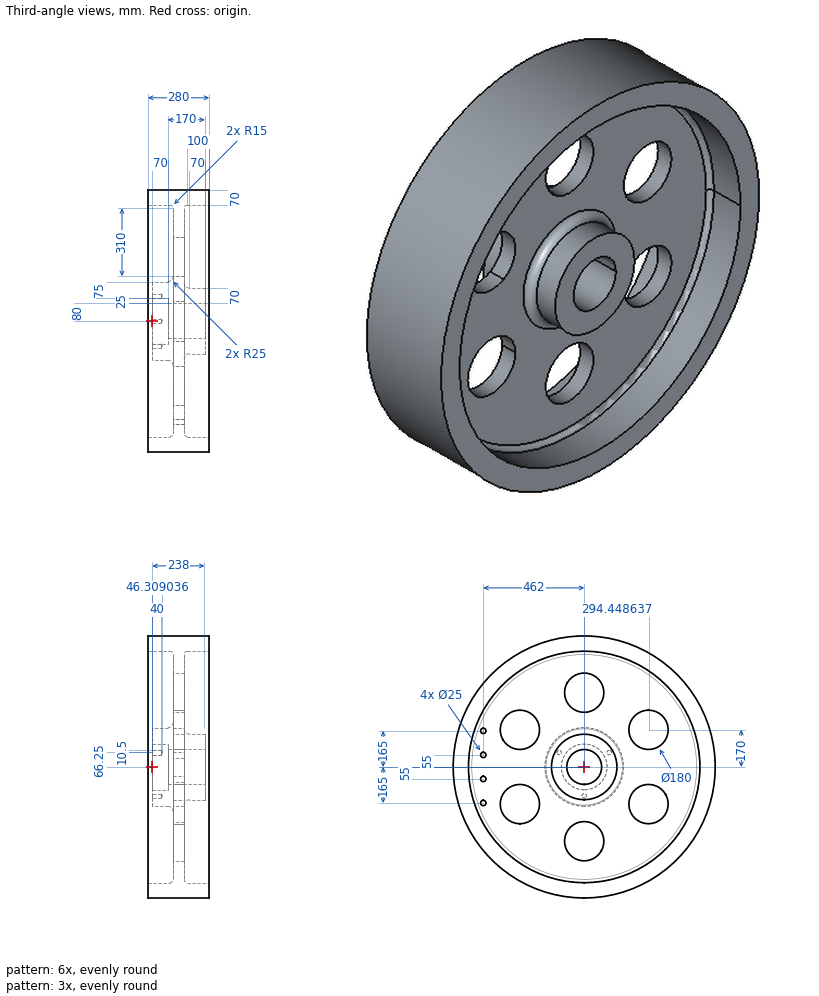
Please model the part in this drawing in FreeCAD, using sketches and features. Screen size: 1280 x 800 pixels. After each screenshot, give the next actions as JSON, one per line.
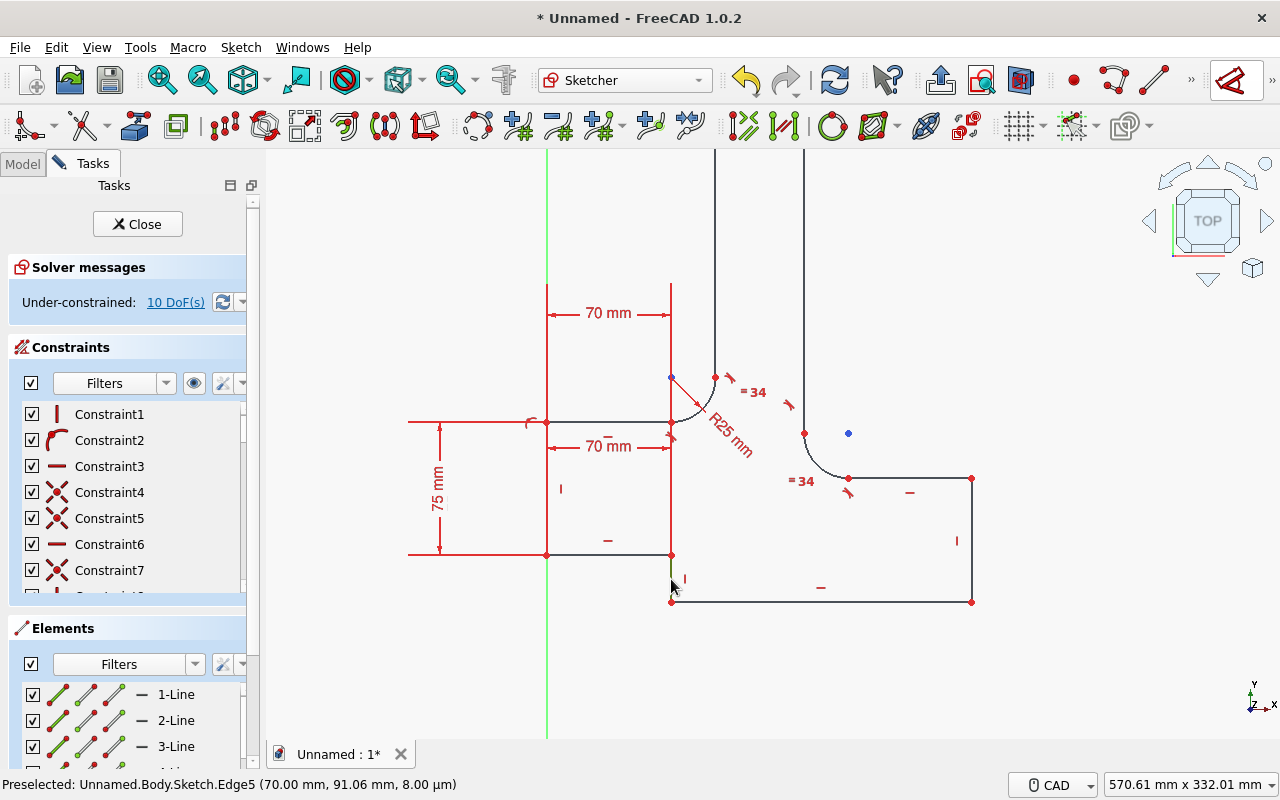
{"action": "key", "text": "i"}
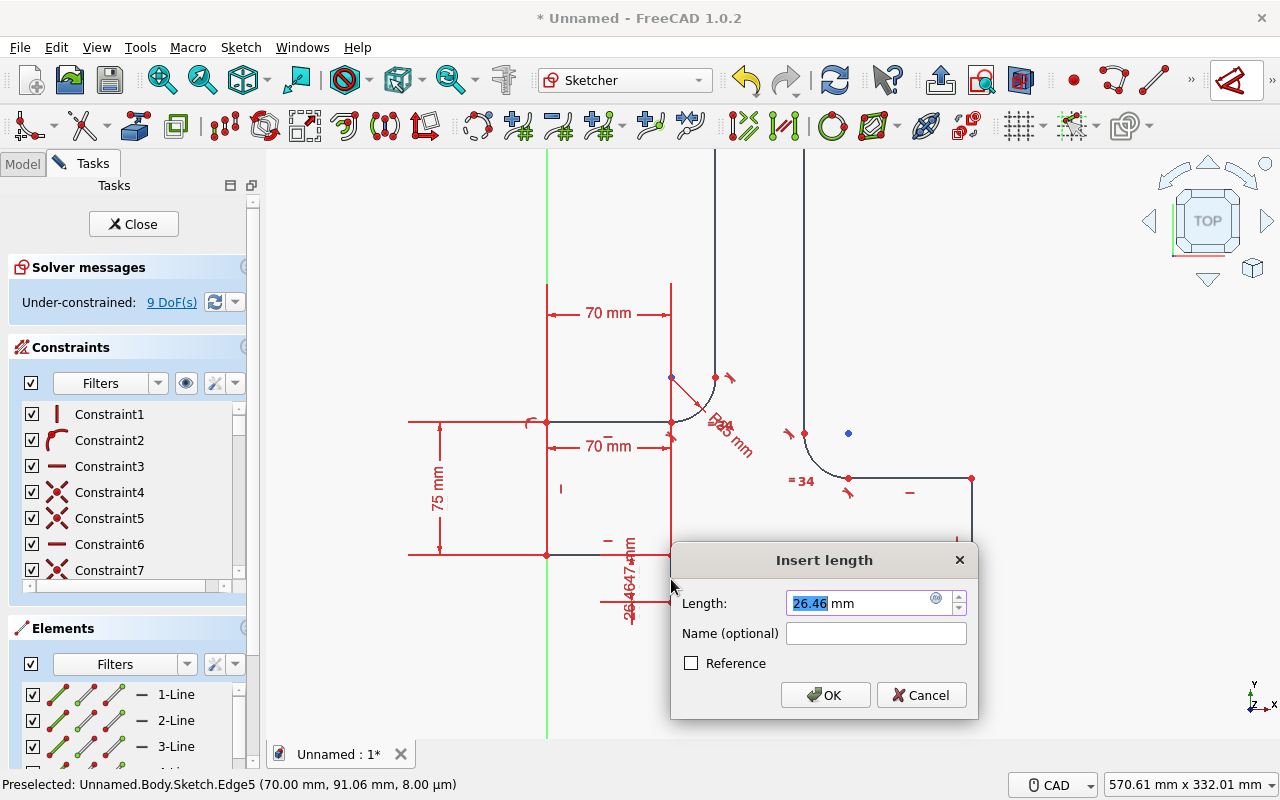
{"action": "type", "text": "25"}
{"action": "key", "text": "Return"}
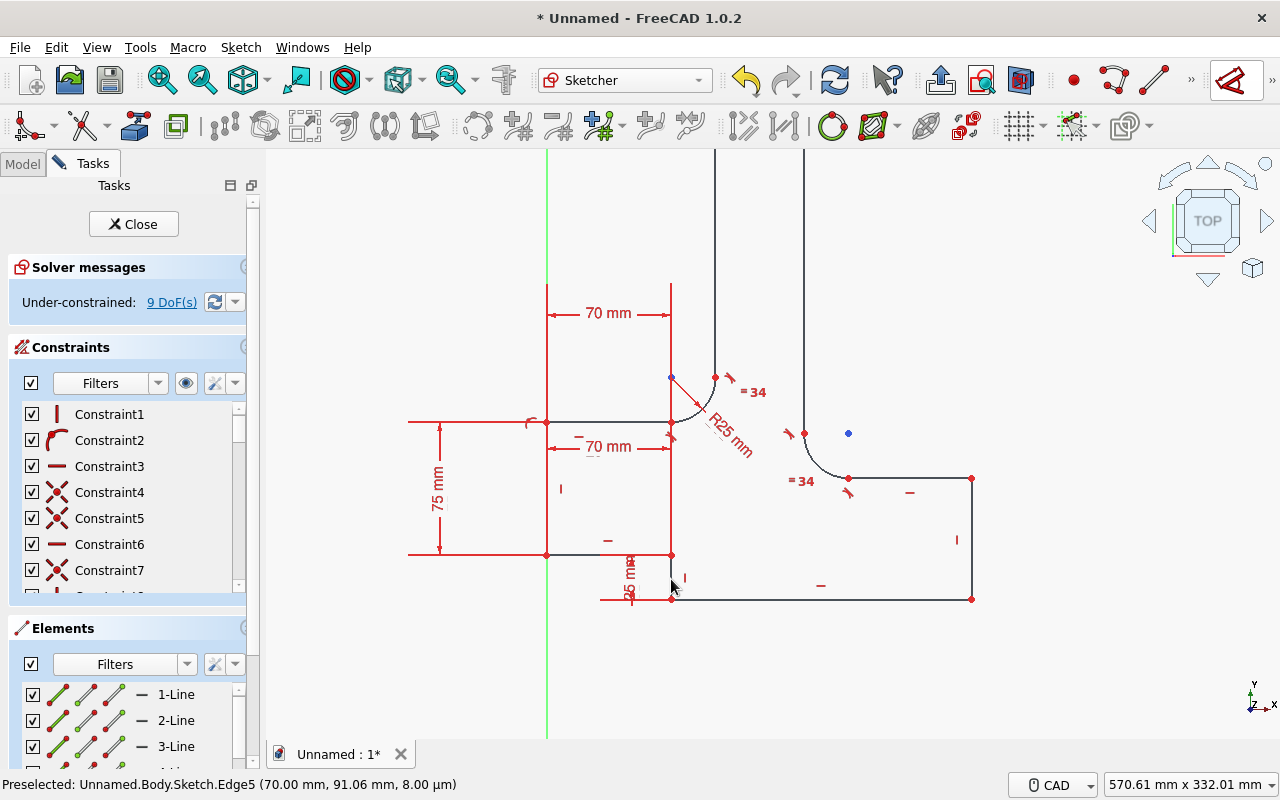
{"action": "left_click", "coordinate": [972, 563]}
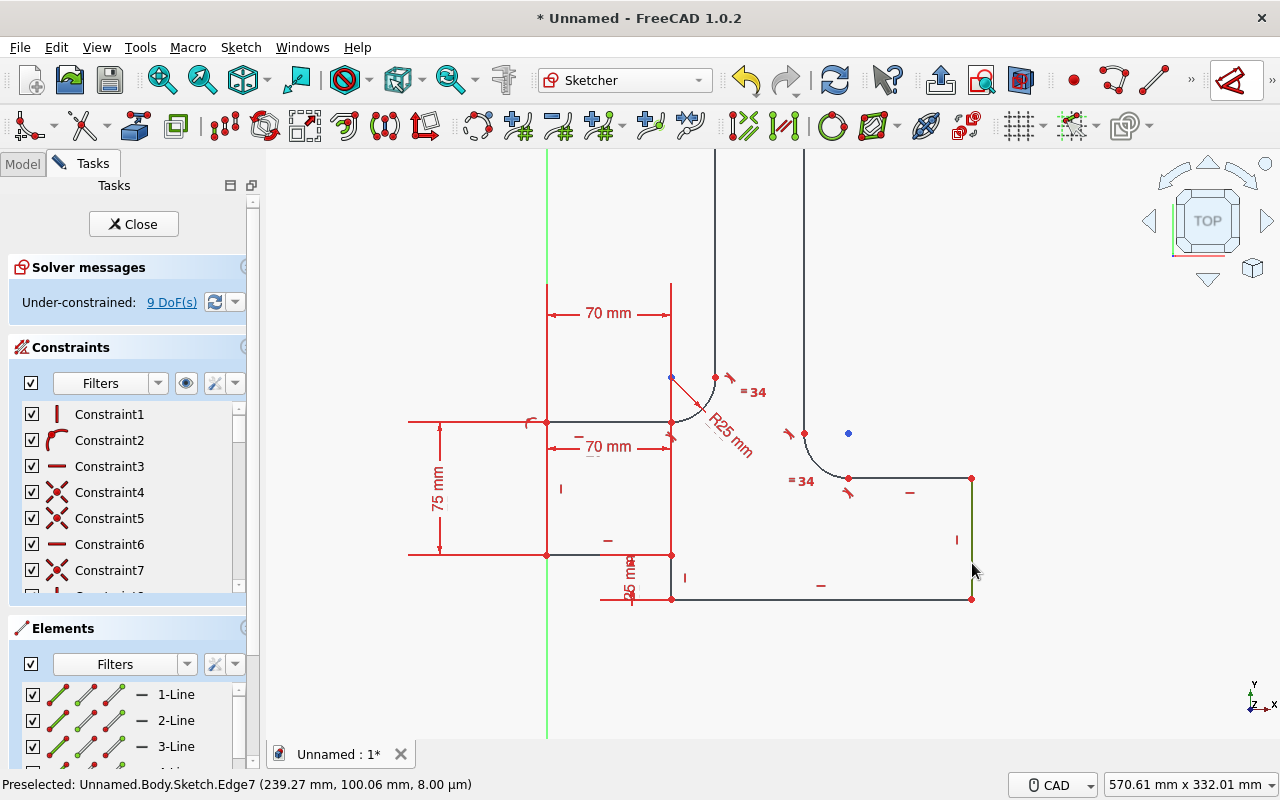
{"action": "left_click", "coordinate": [1258, 80]}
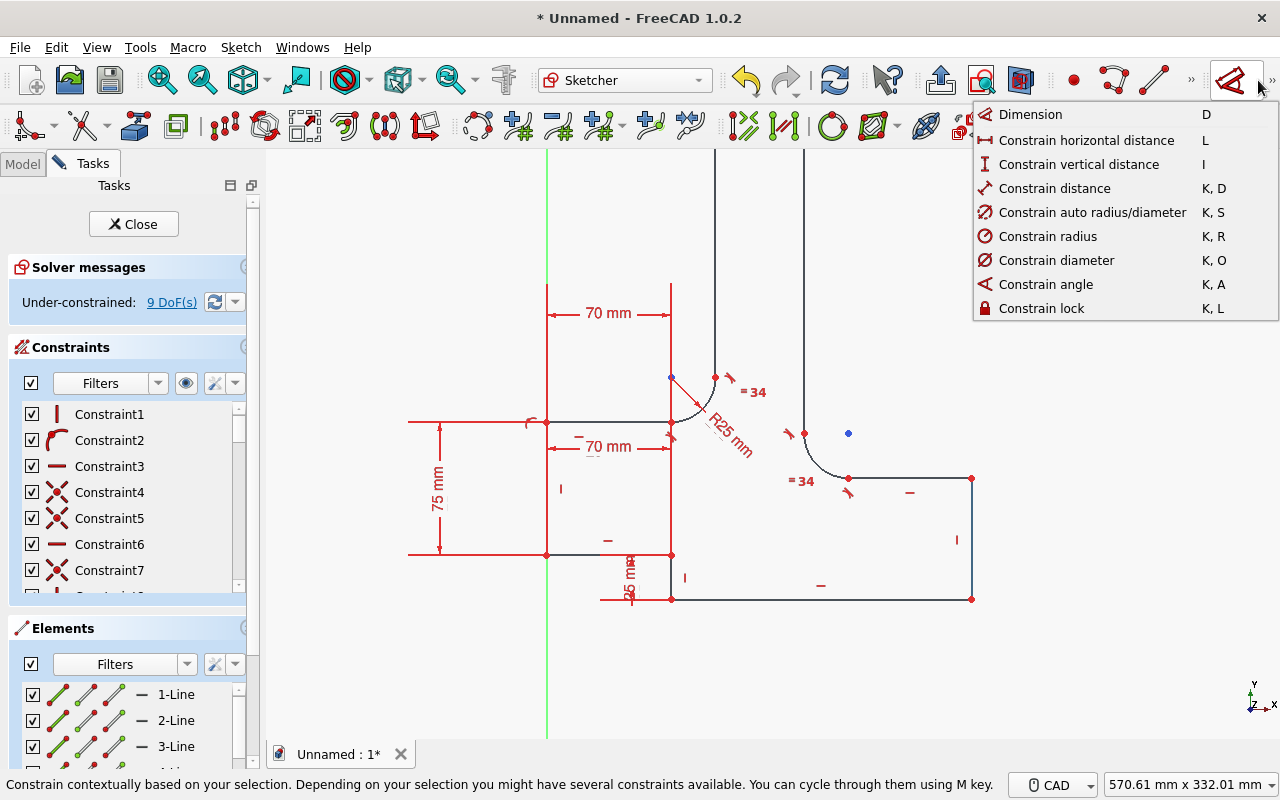
{"action": "left_click", "coordinate": [1126, 164]}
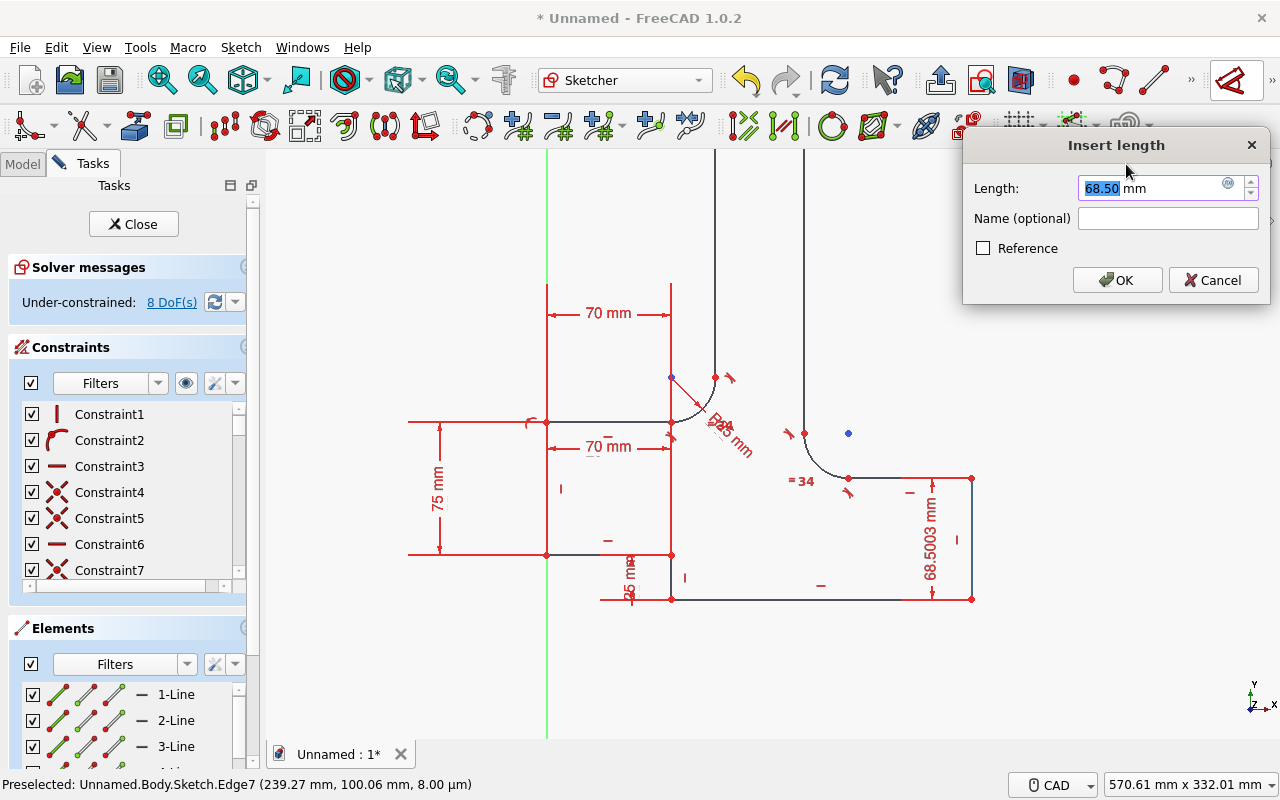
{"action": "type", "text": "70"}
{"action": "key", "text": "Return"}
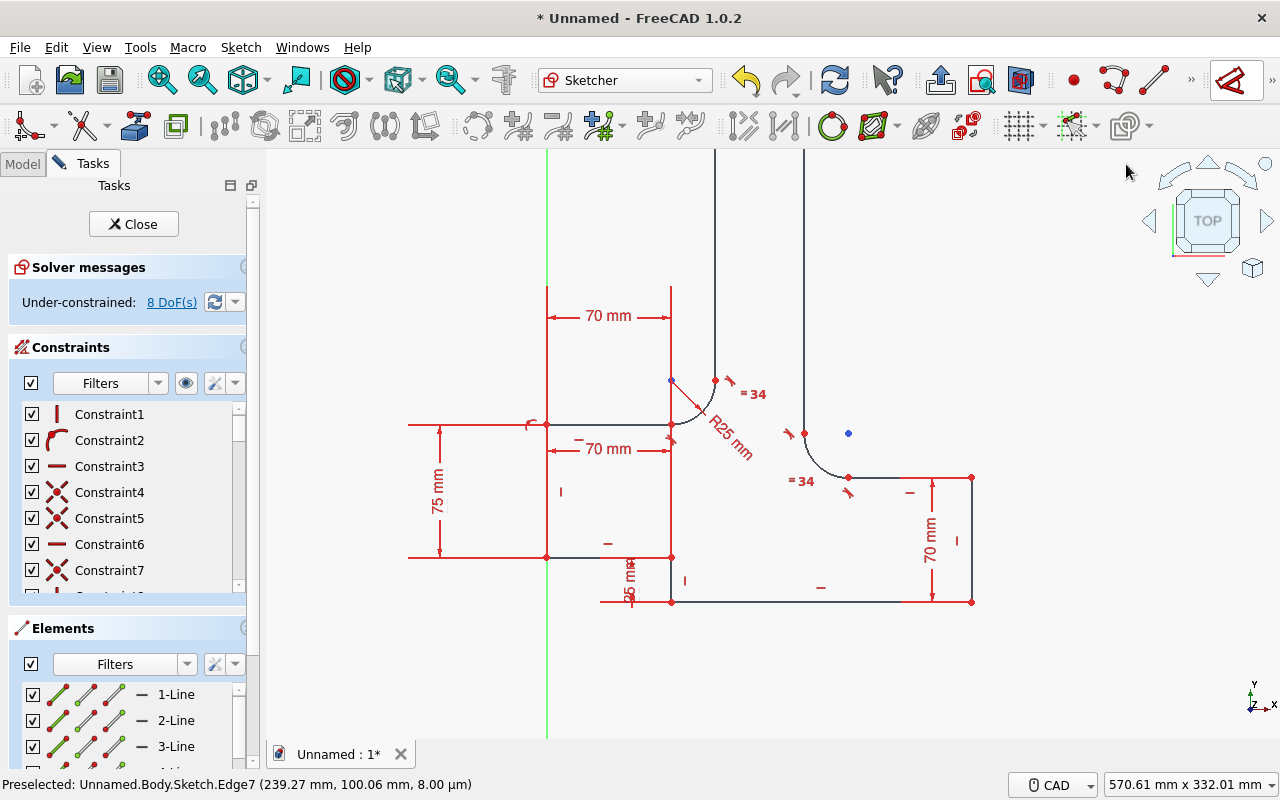
{"action": "left_click", "coordinate": [935, 478]}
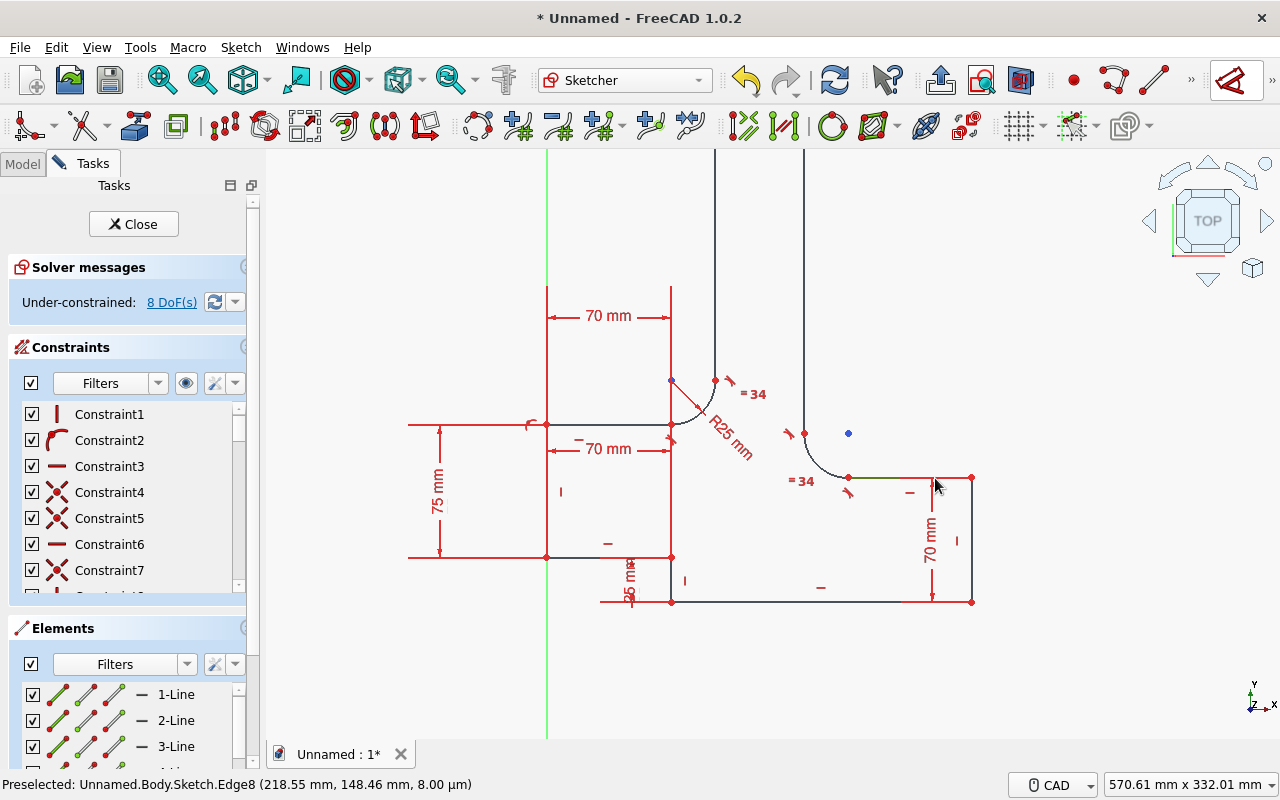
{"action": "key", "text": "l"}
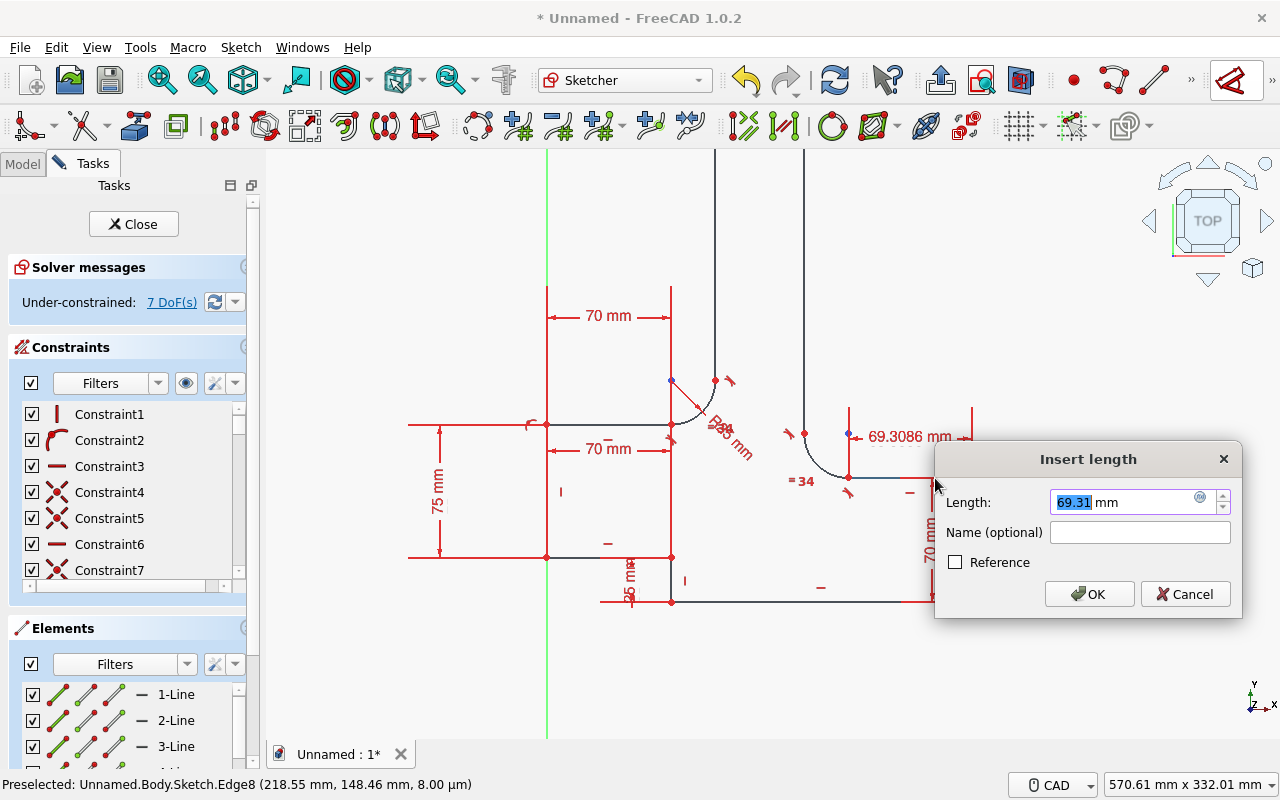
{"action": "type", "text": "70"}
{"action": "key", "text": "Return"}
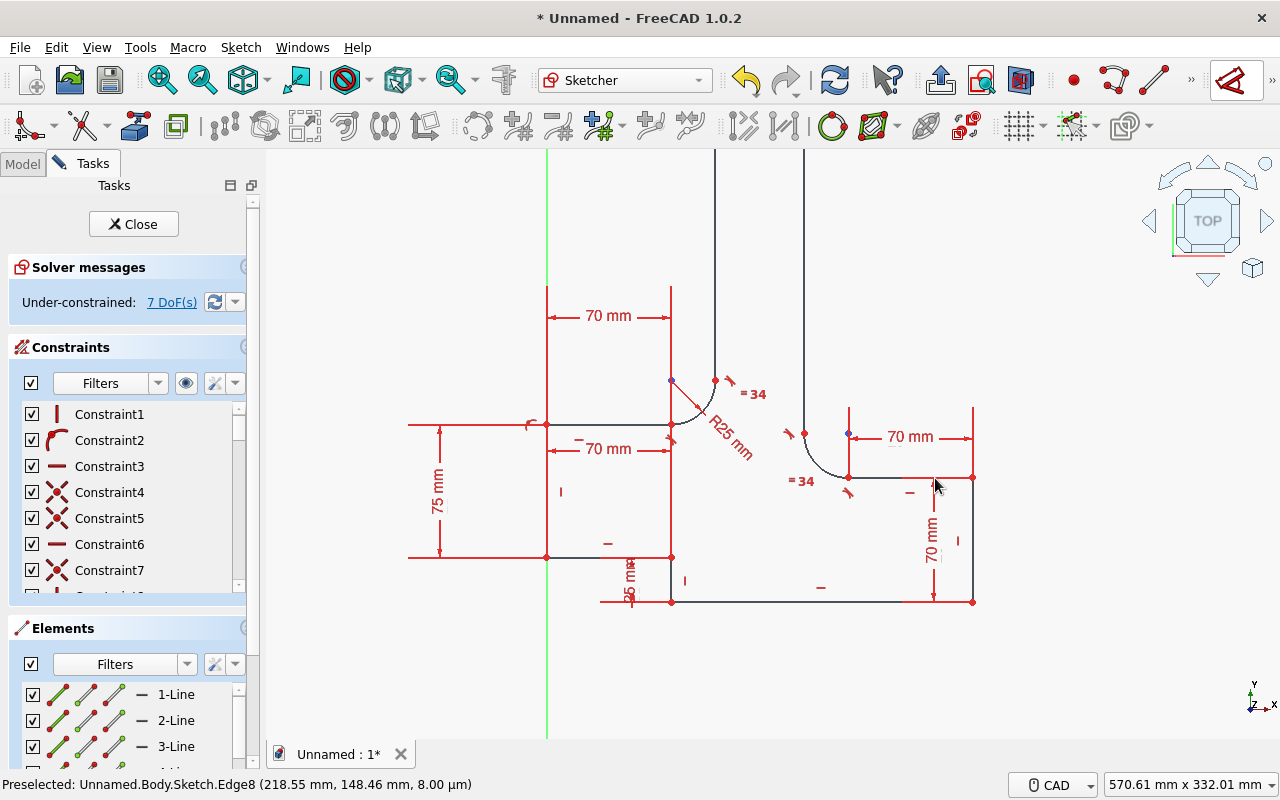
{"action": "scroll", "coordinate": [672, 581], "scroll_direction": "down", "scroll_amount": 5}